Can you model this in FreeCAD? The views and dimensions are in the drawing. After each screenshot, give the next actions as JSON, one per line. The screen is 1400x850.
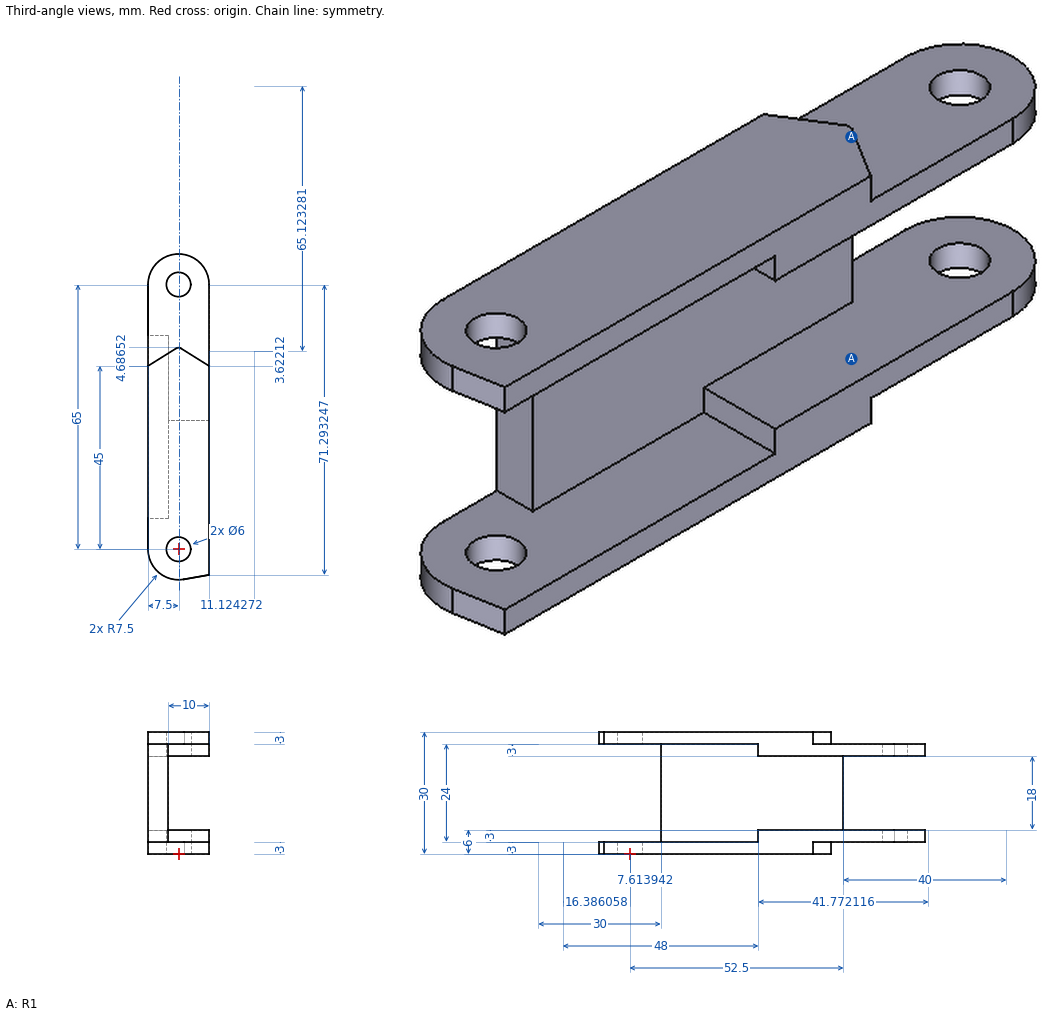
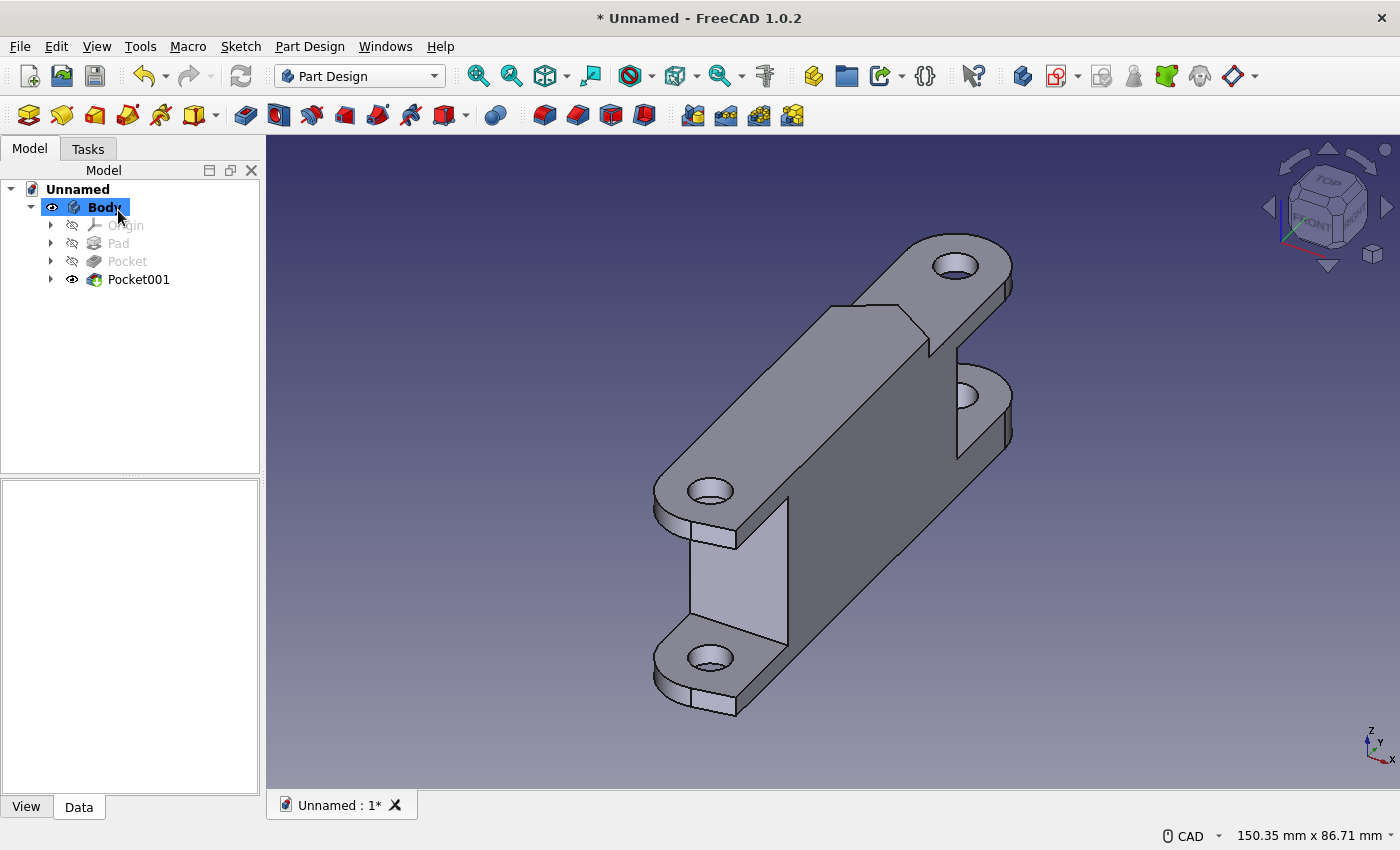
{"action": "key", "text": "5"}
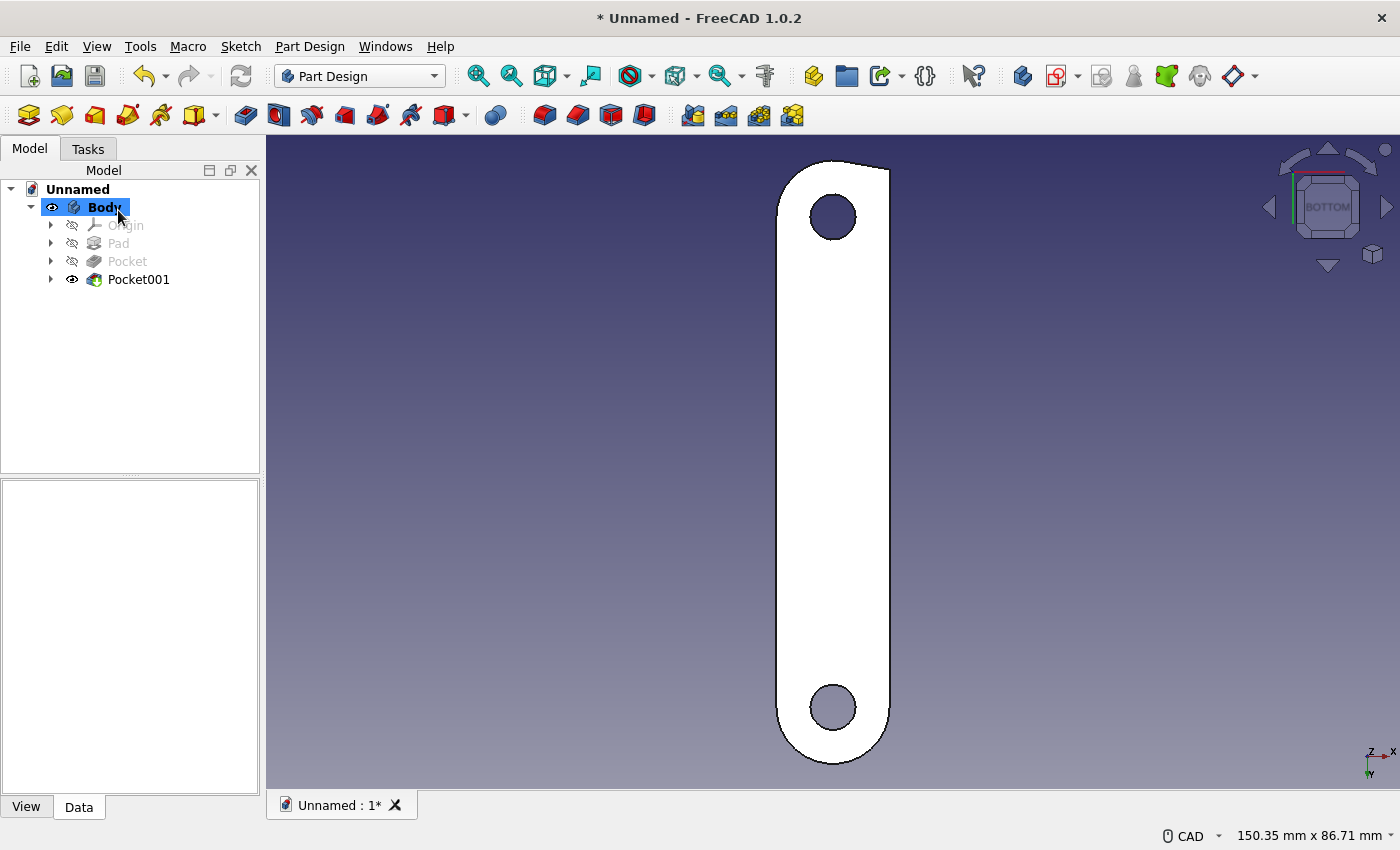
{"action": "left_click", "coordinate": [833, 547]}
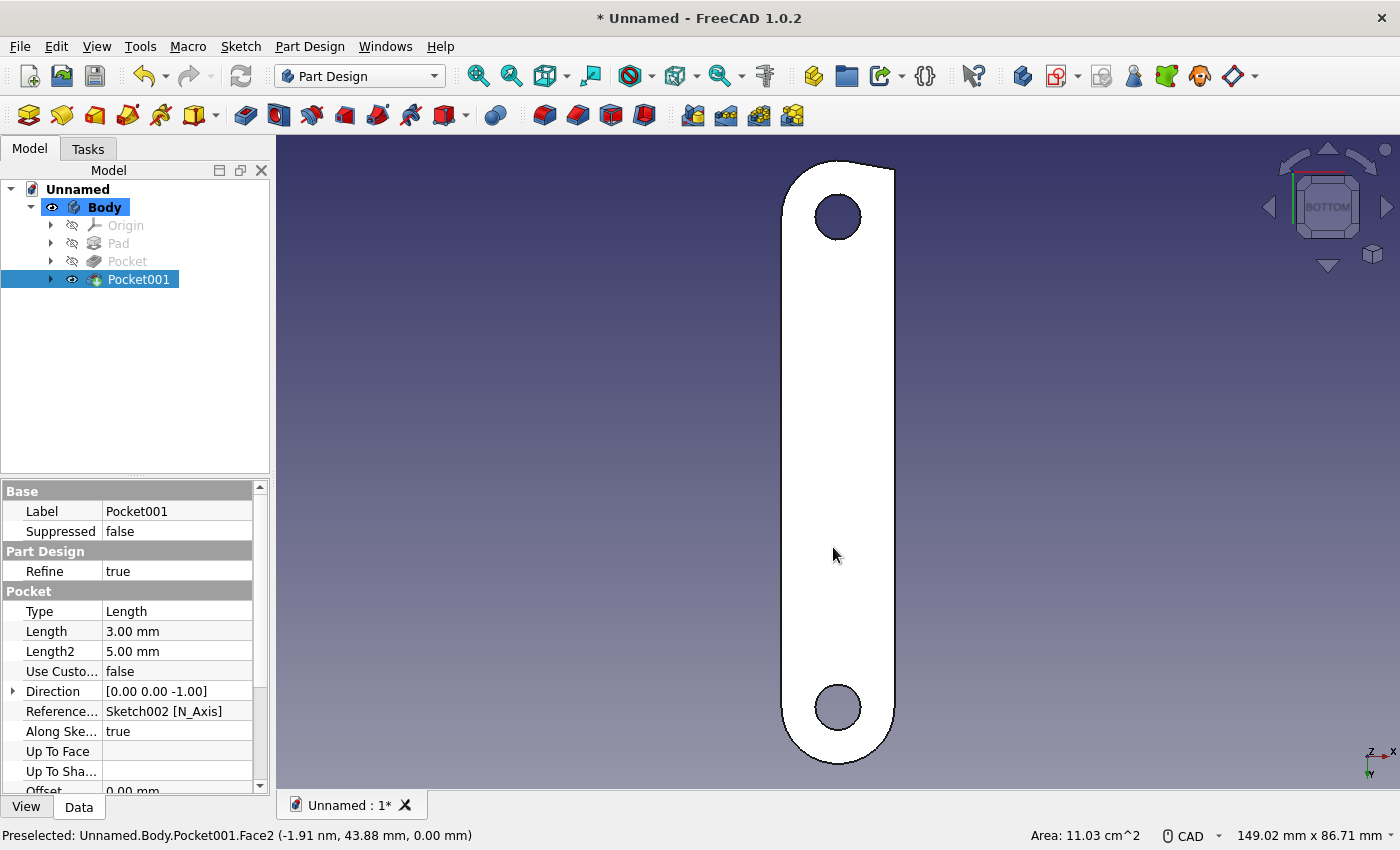
{"action": "left_click", "coordinate": [1056, 76]}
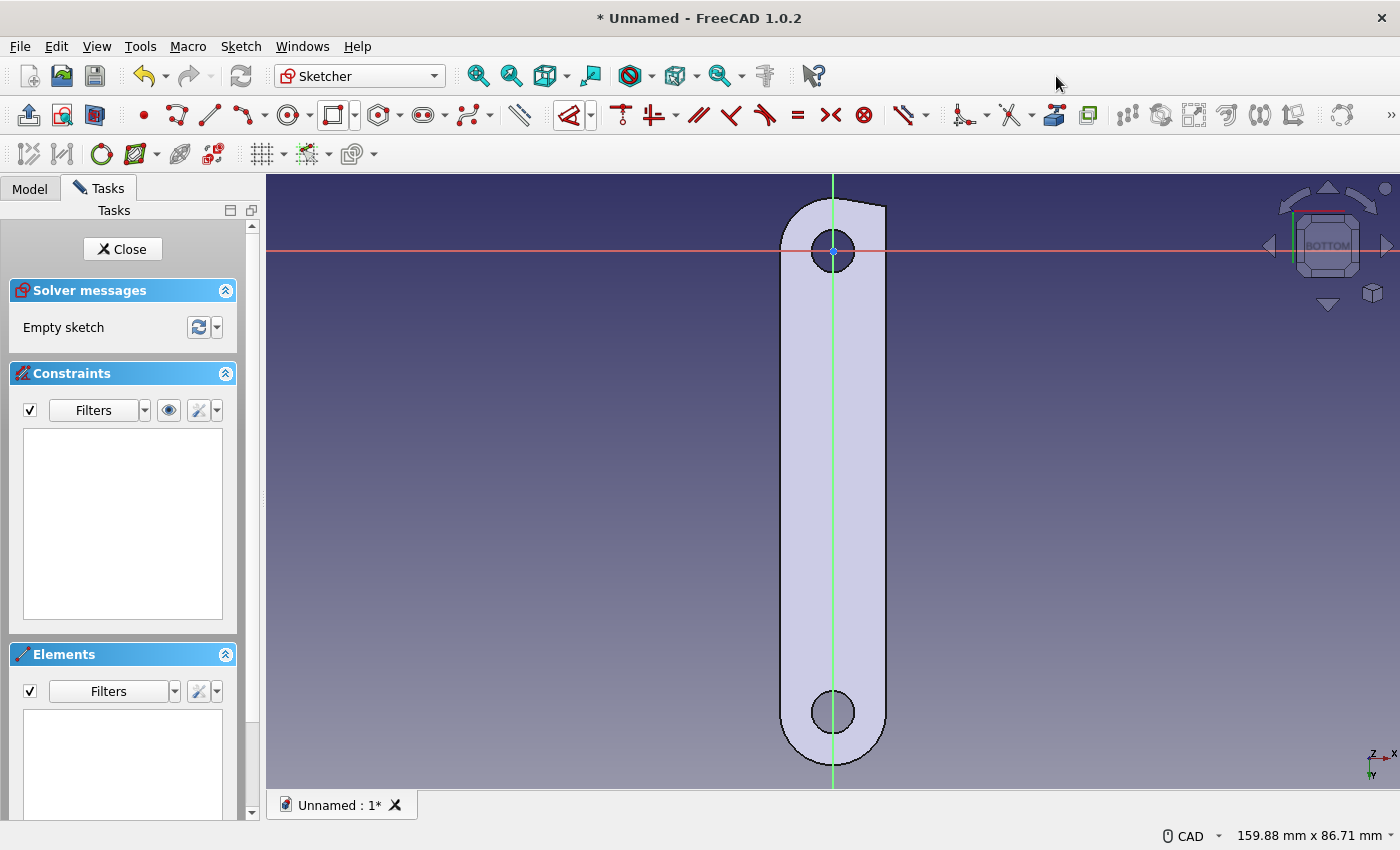
{"action": "scroll", "coordinate": [709, 340], "scroll_direction": "down", "scroll_amount": 4}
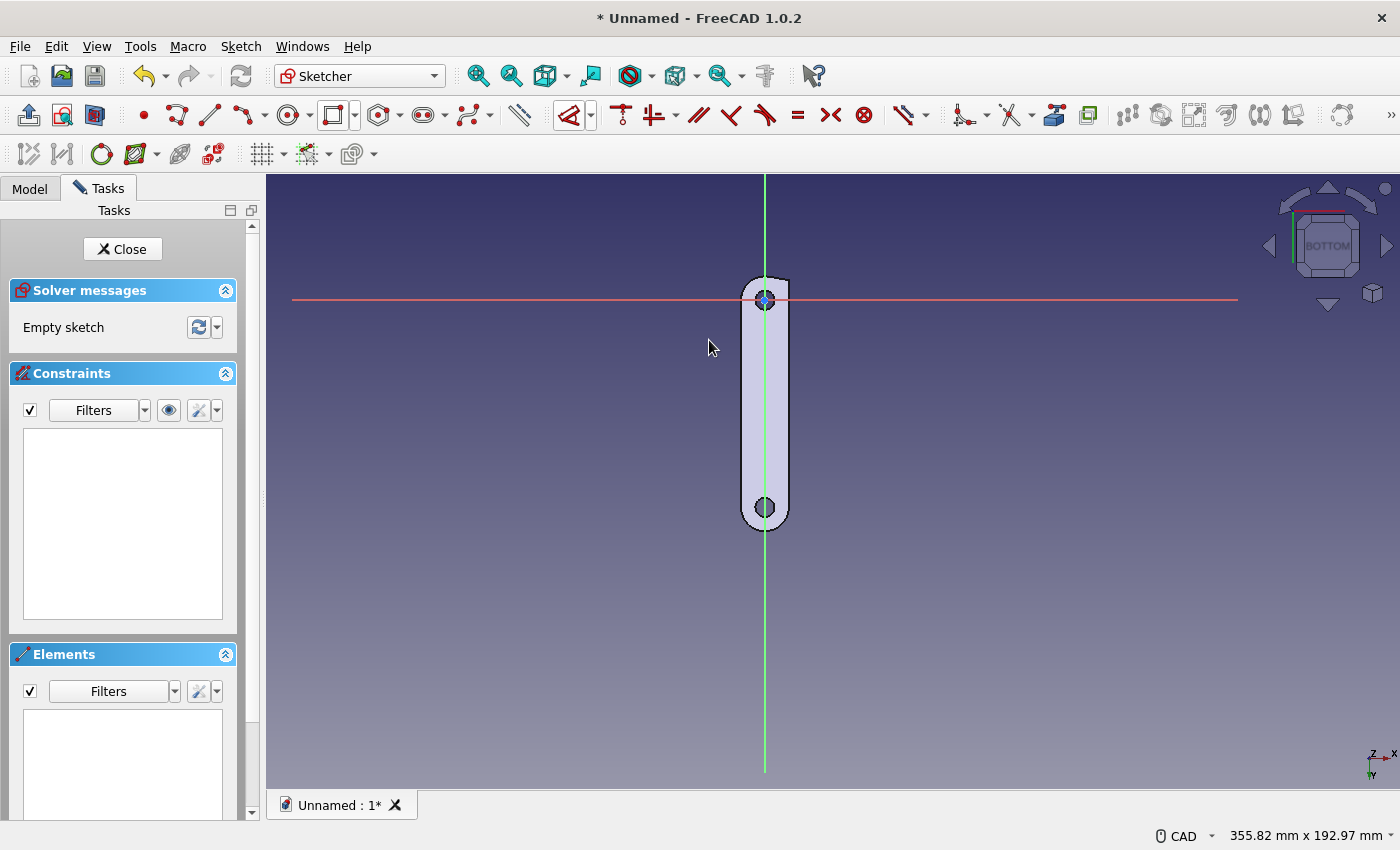
{"action": "key", "text": "g m"}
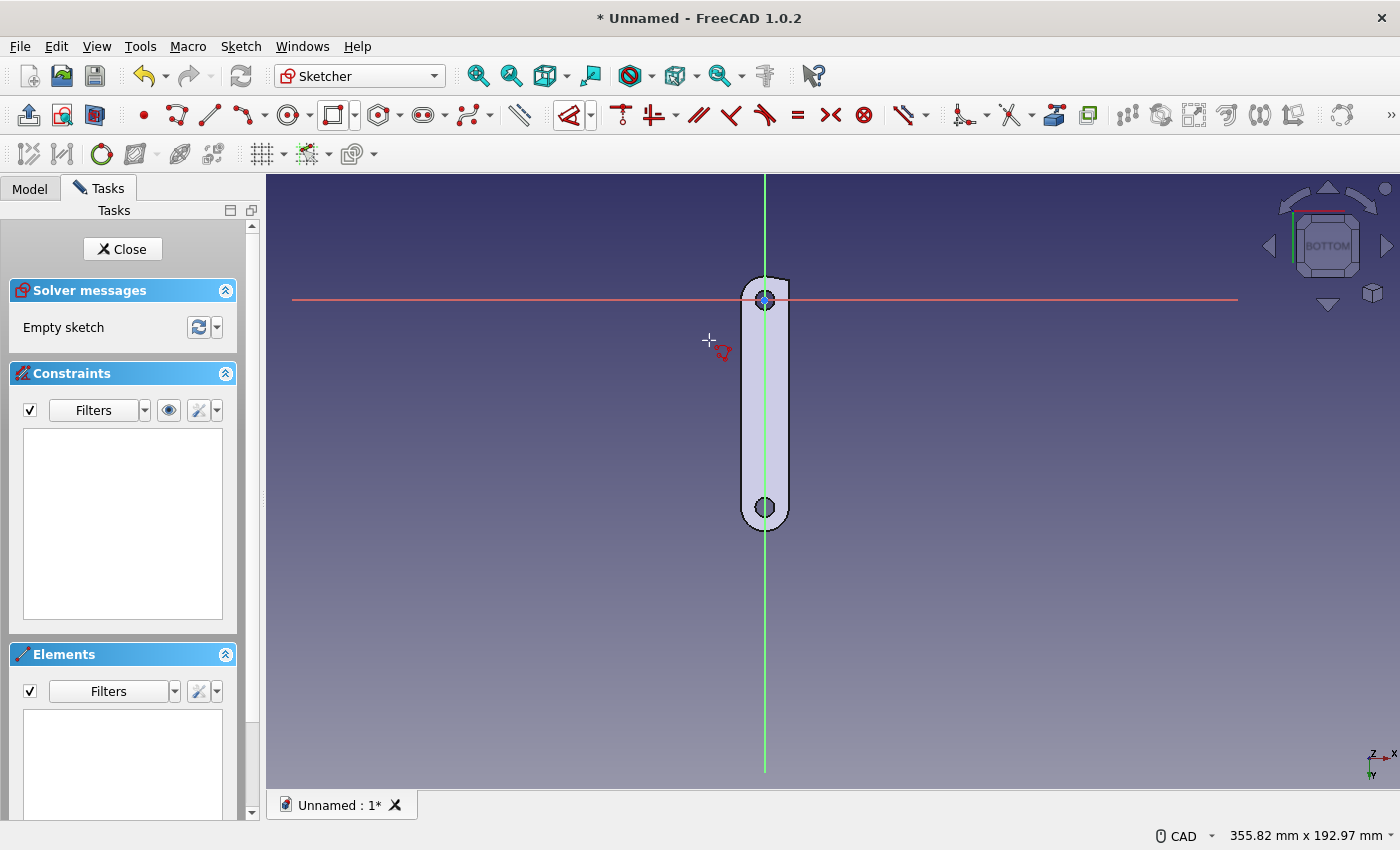
{"action": "left_click", "coordinate": [741, 444]}
{"action": "left_click", "coordinate": [765, 459]}
{"action": "left_click", "coordinate": [789, 444]}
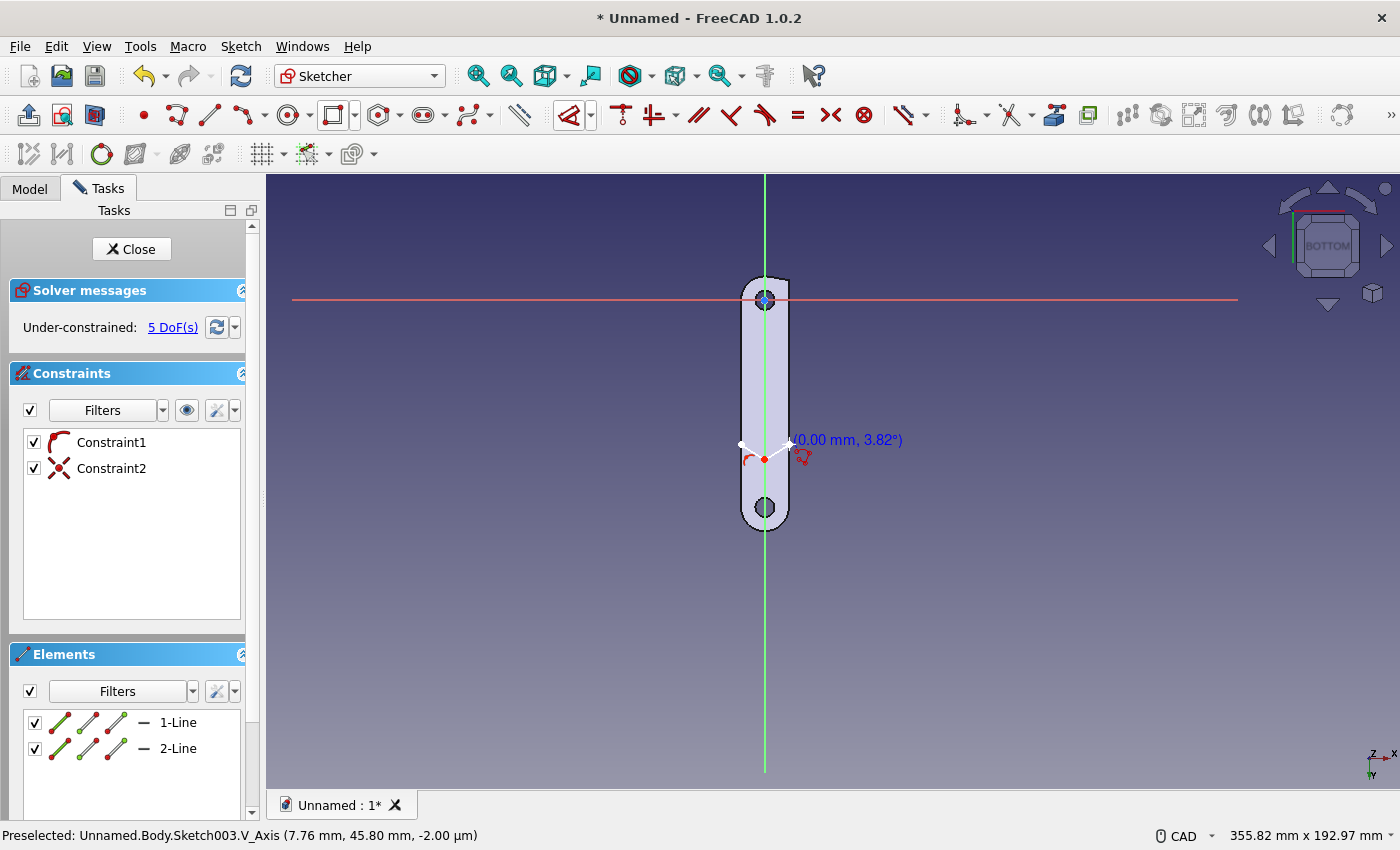
{"action": "scroll", "coordinate": [789, 455], "scroll_direction": "up", "scroll_amount": 3}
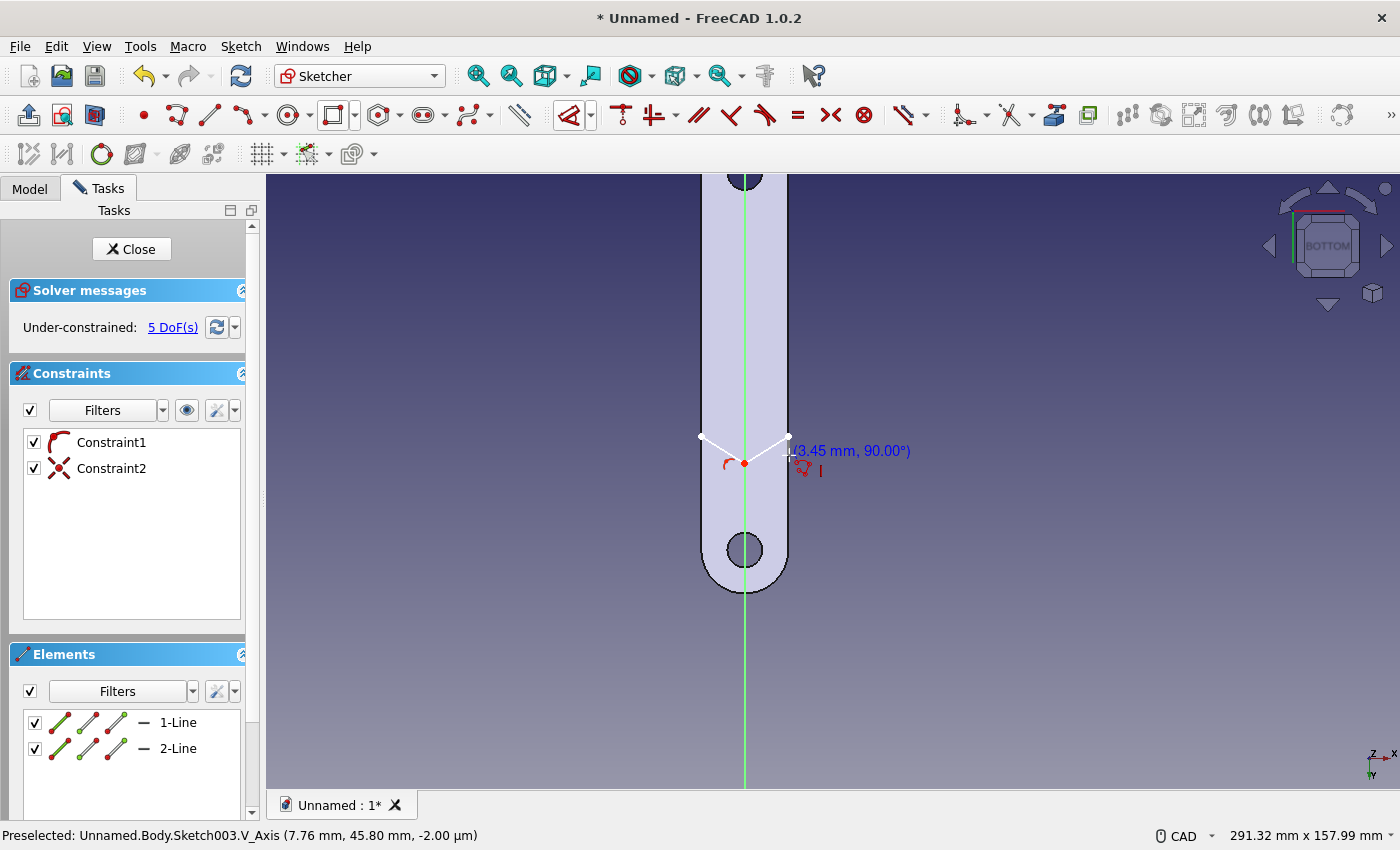
{"action": "left_click", "coordinate": [789, 455]}
{"action": "left_click", "coordinate": [853, 455]}